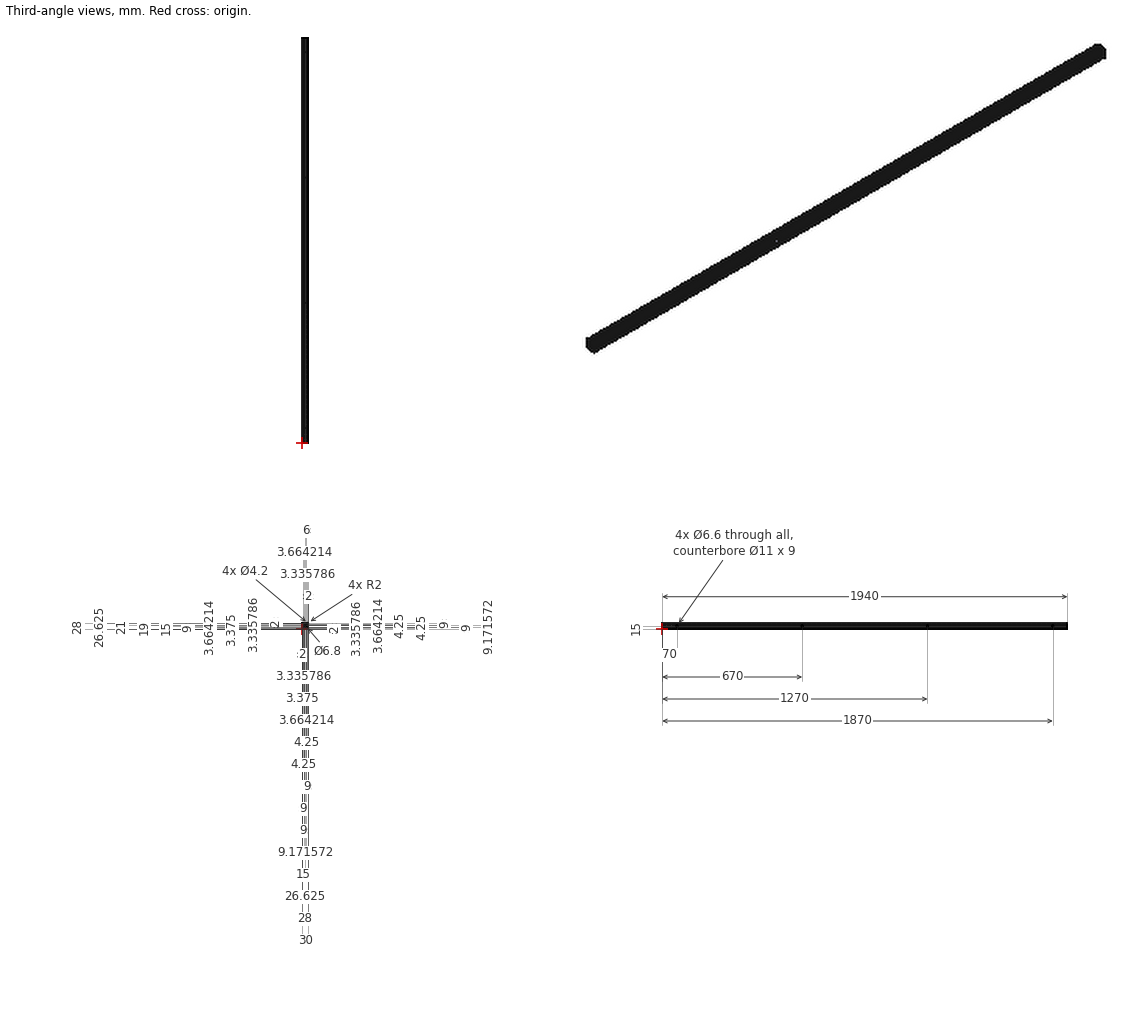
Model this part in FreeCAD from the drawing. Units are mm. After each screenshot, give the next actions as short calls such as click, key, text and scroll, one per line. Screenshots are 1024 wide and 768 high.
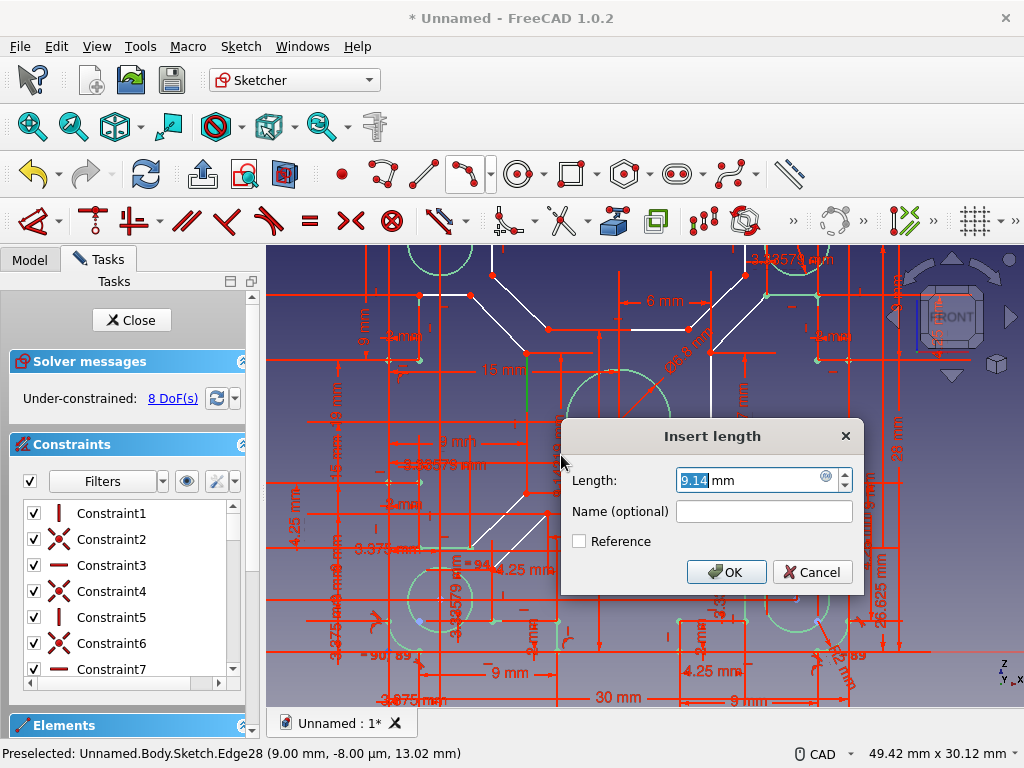
text(9.171572)
key(Return)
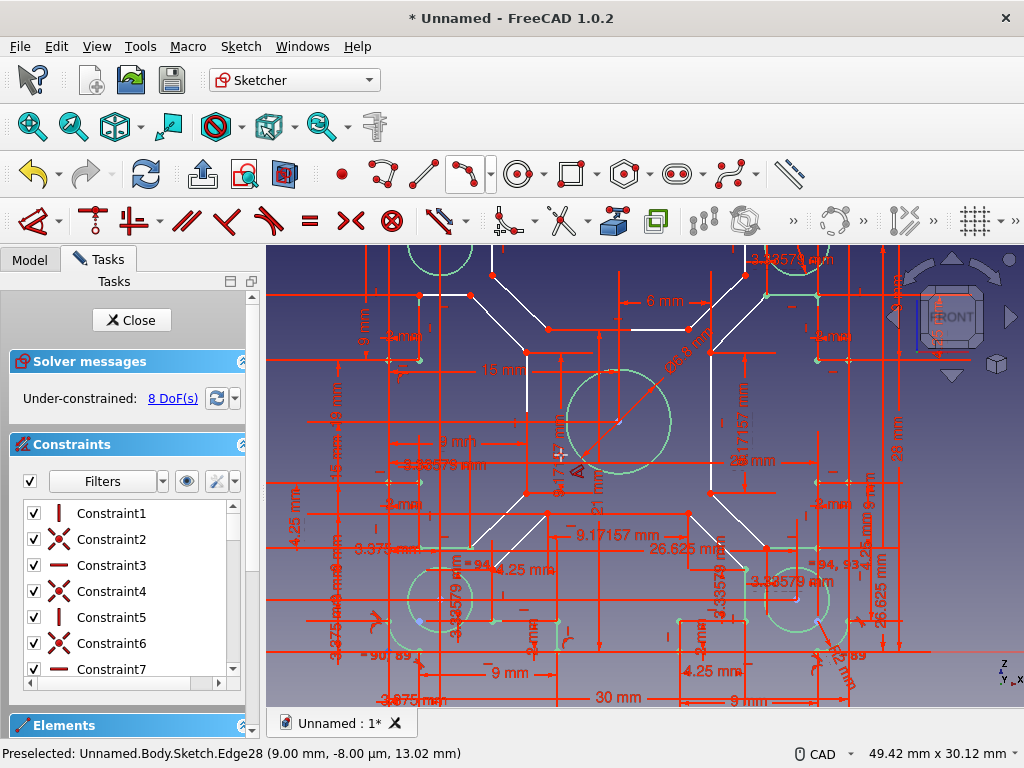
click(455, 295)
click(433, 377)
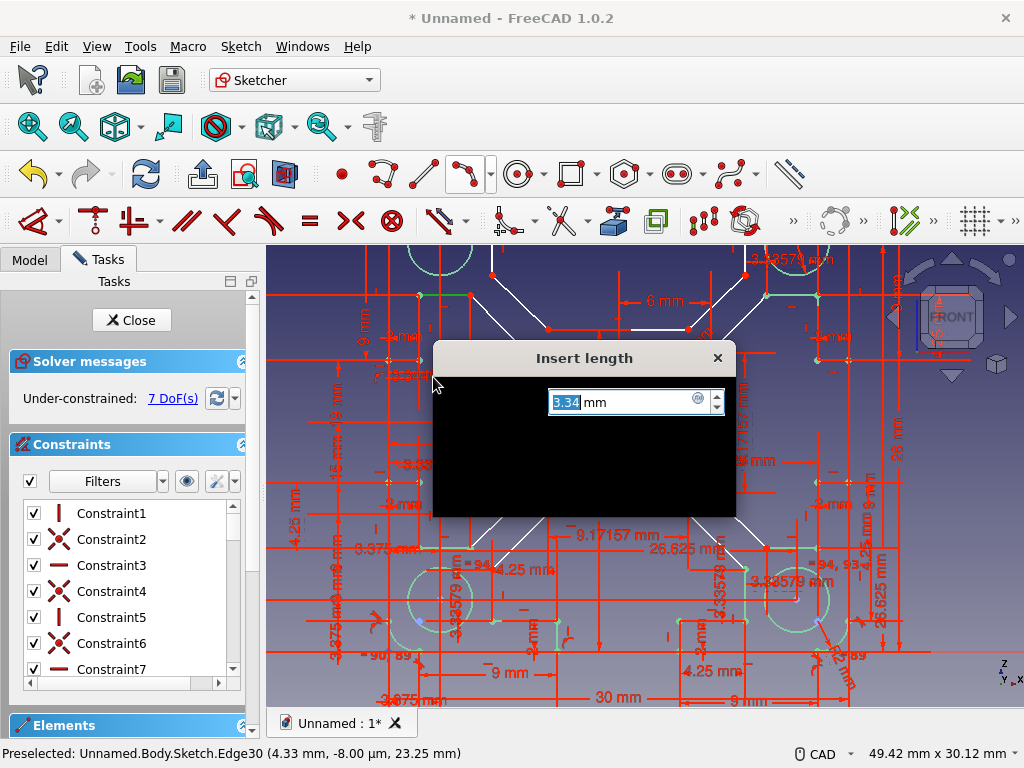
text(3.335786)
key(Return)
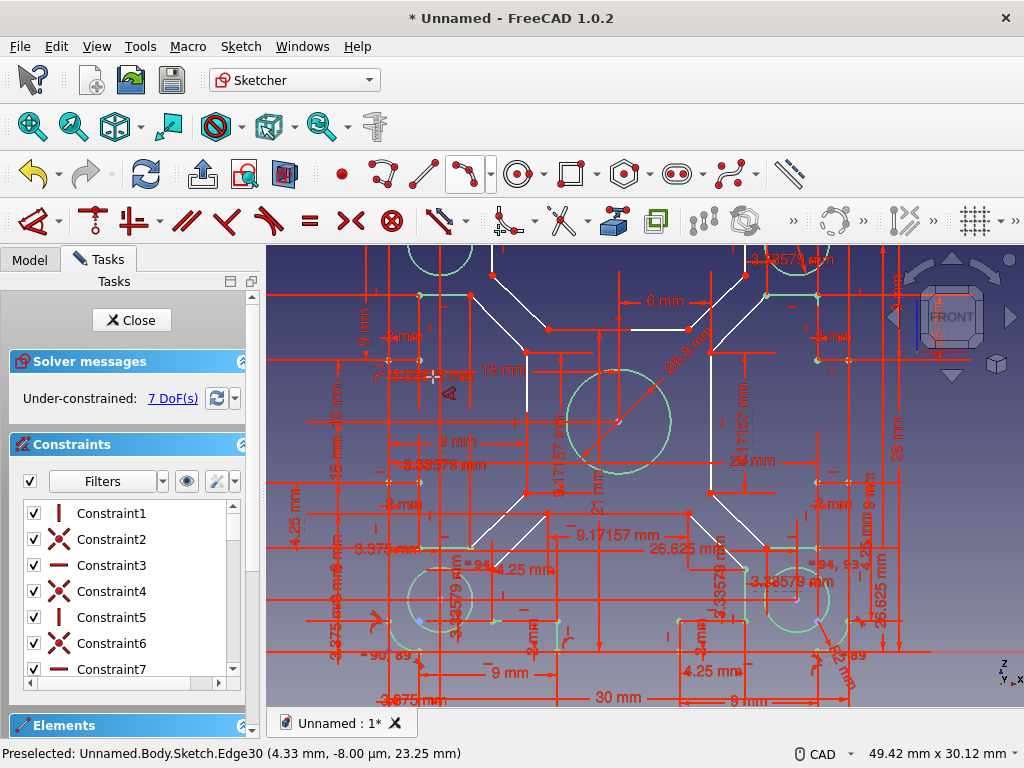
scroll(491, 587, down, 2)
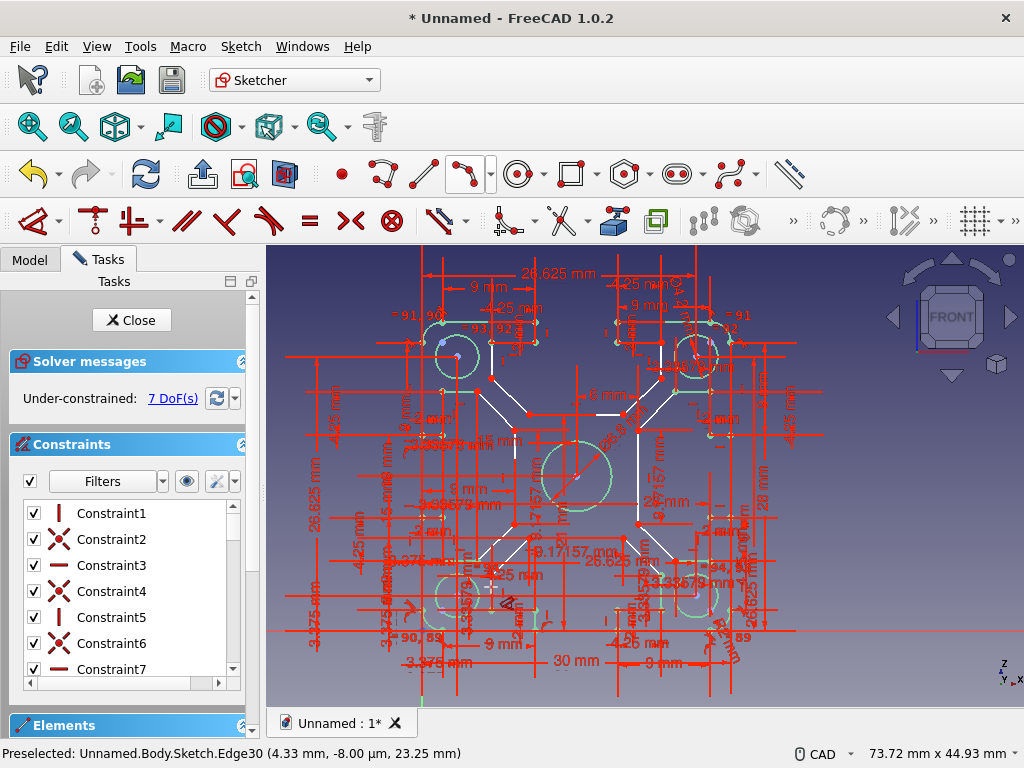
scroll(492, 353, up, 2)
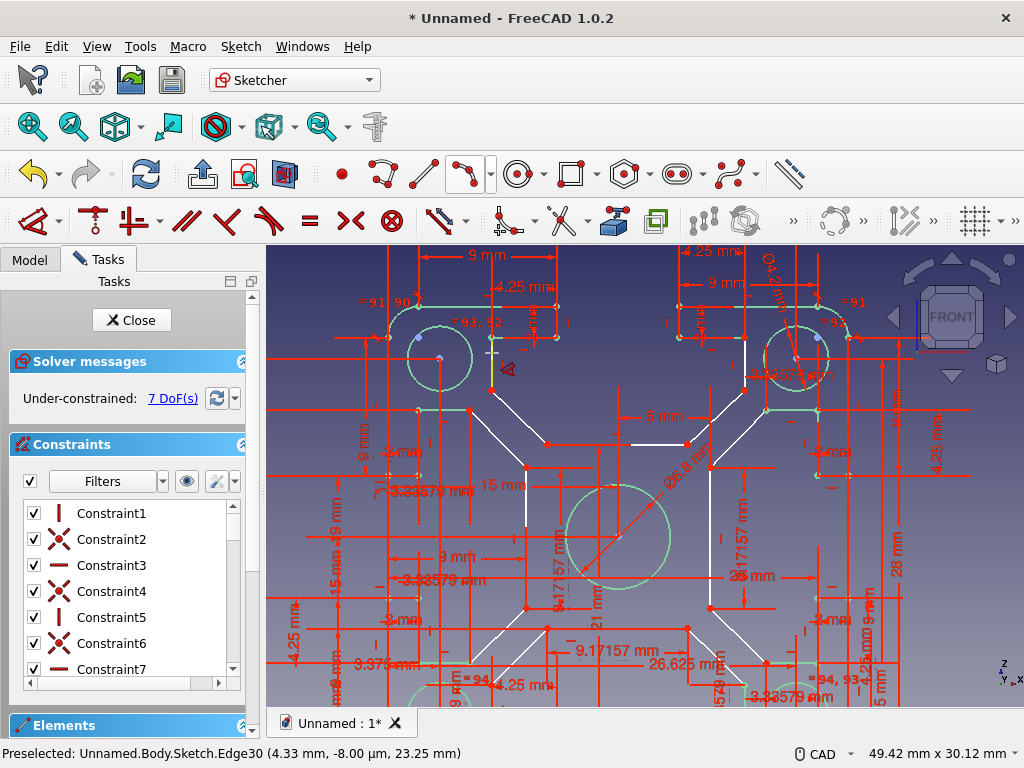
click(492, 354)
click(458, 364)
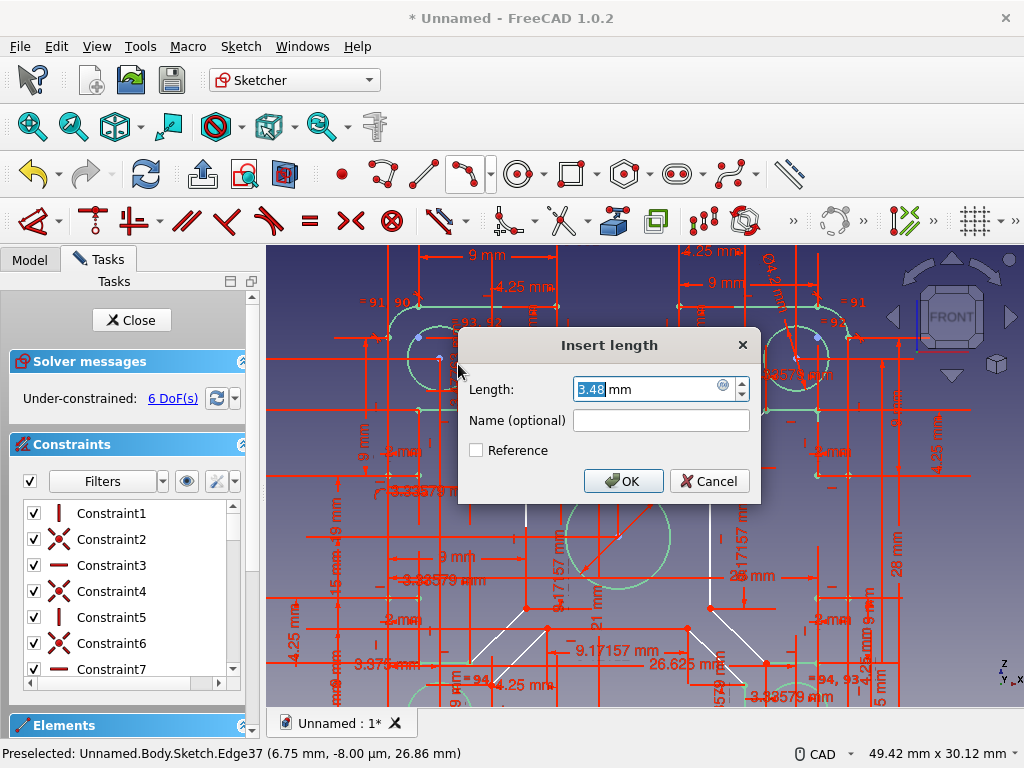
text(3.335786)
key(Return)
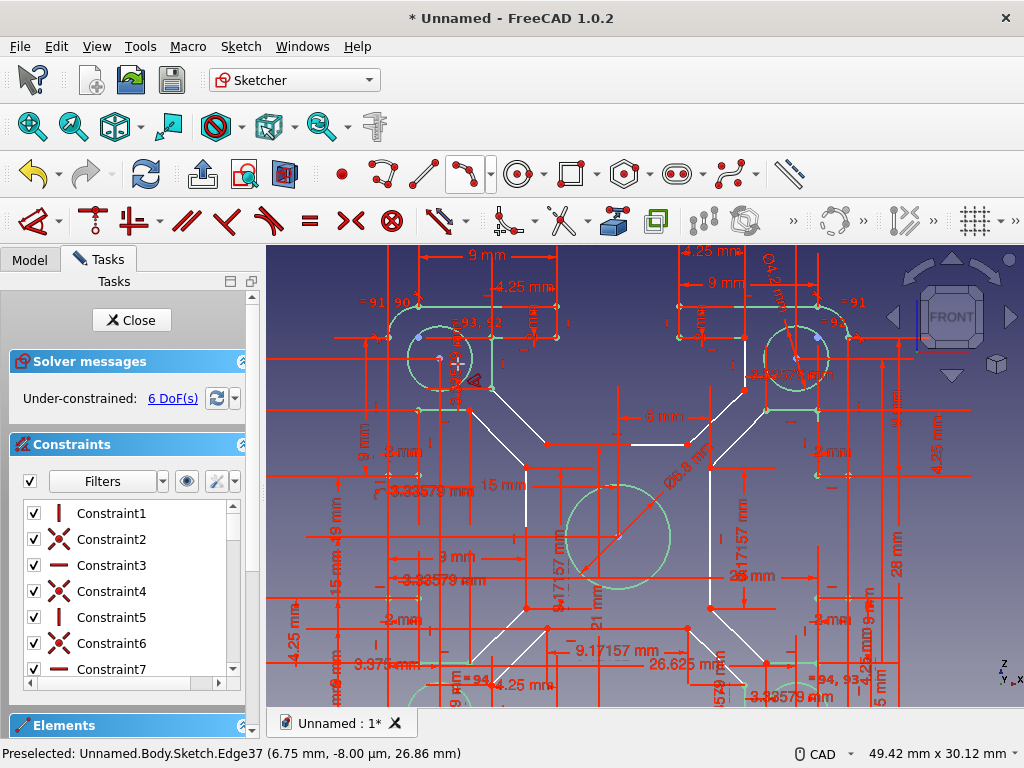
click(590, 445)
click(585, 411)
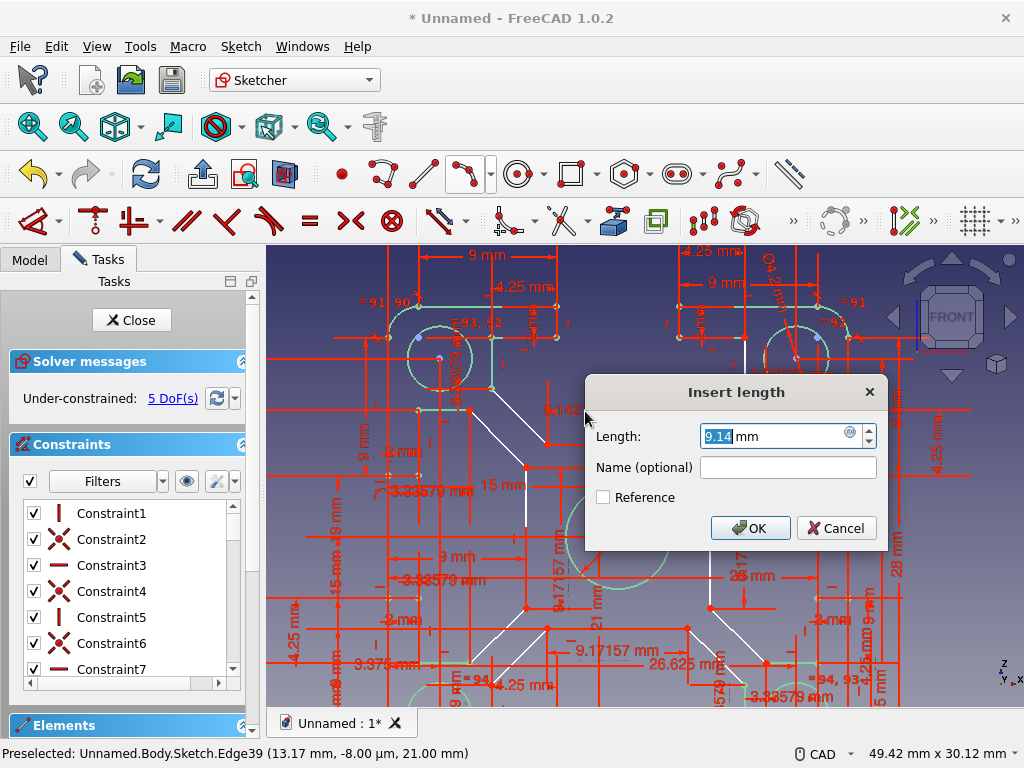
text(9.171572)
key(Return)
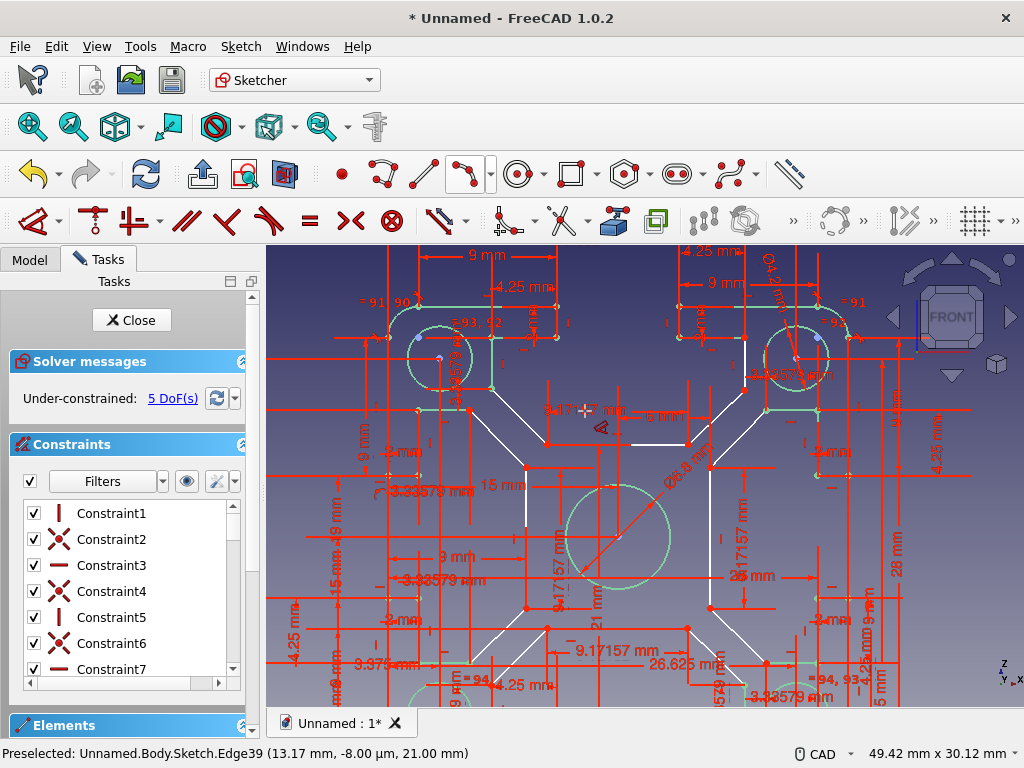
click(745, 375)
click(779, 352)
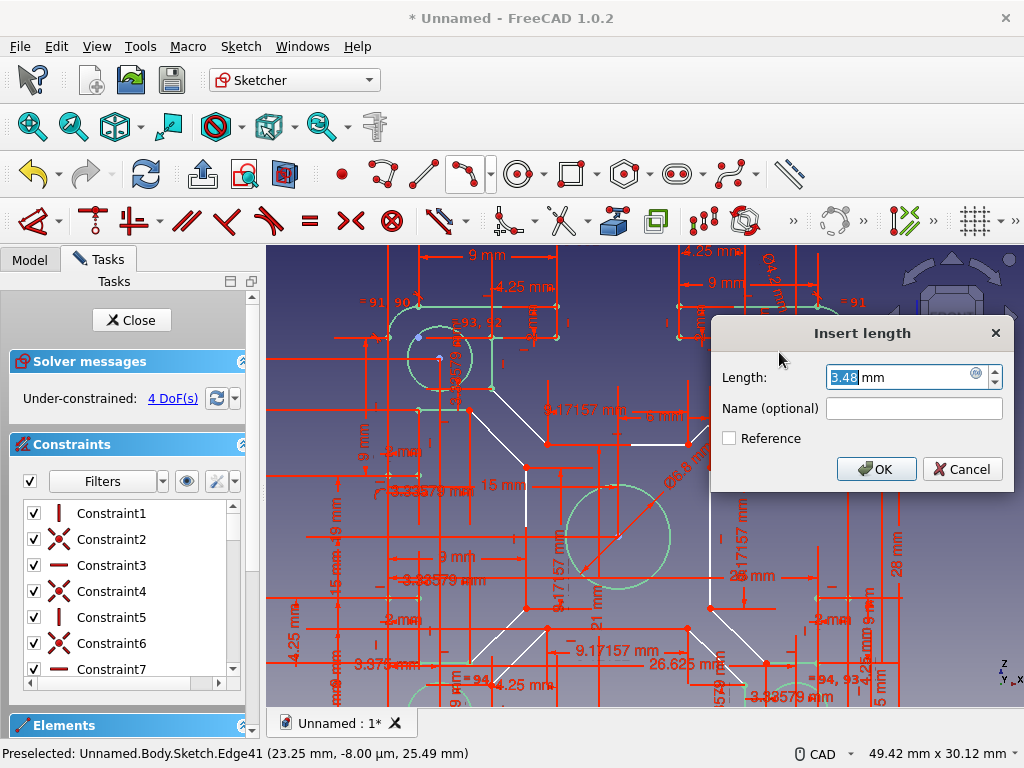
text(3.335786)
key(Return)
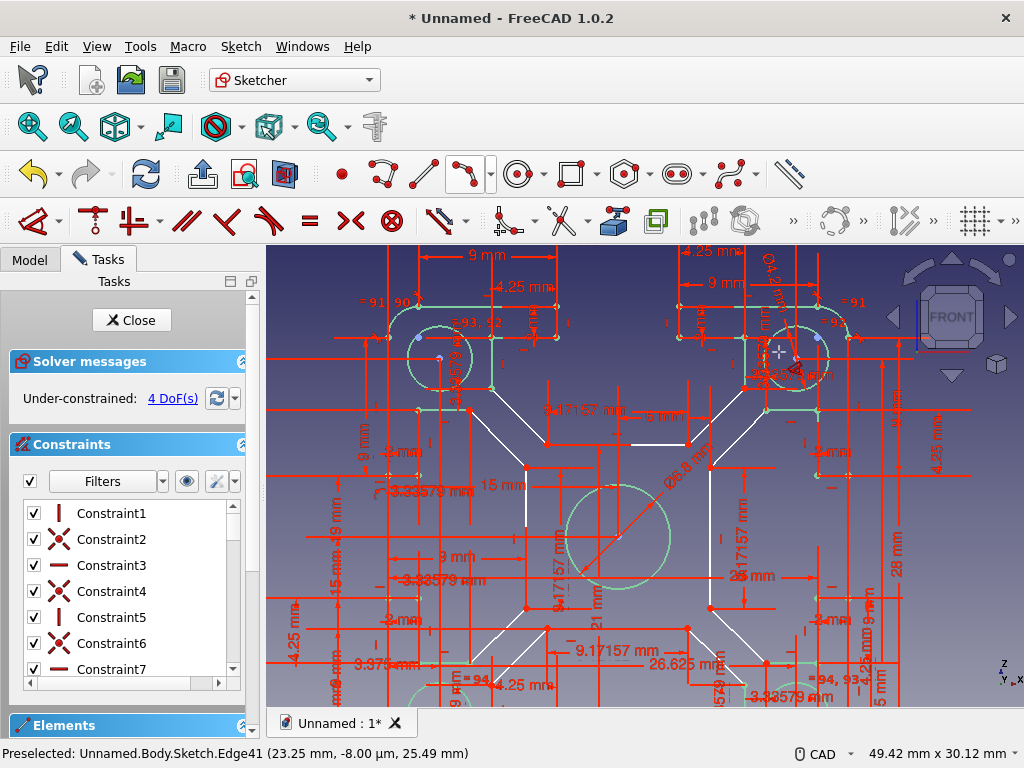
click(749, 428)
click(800, 426)